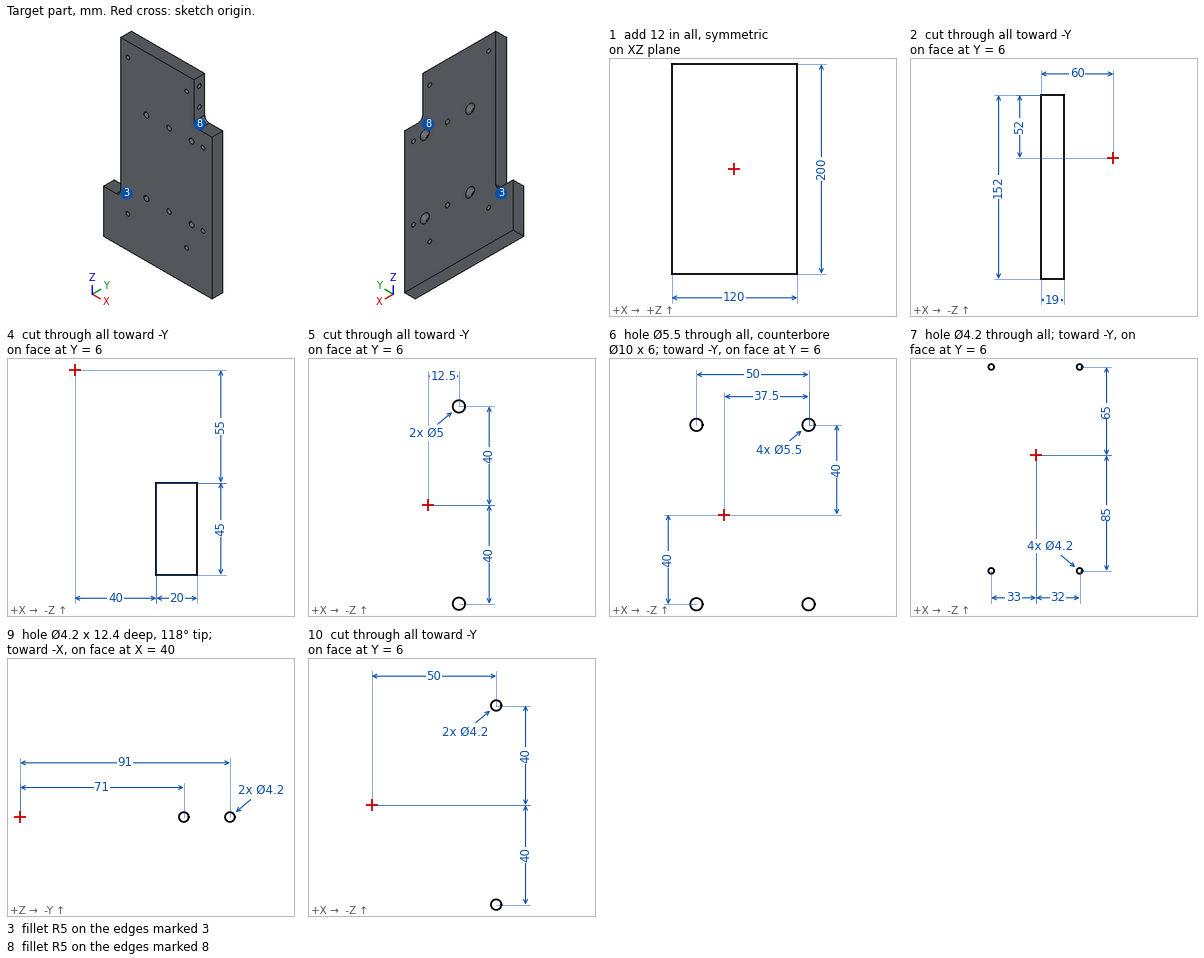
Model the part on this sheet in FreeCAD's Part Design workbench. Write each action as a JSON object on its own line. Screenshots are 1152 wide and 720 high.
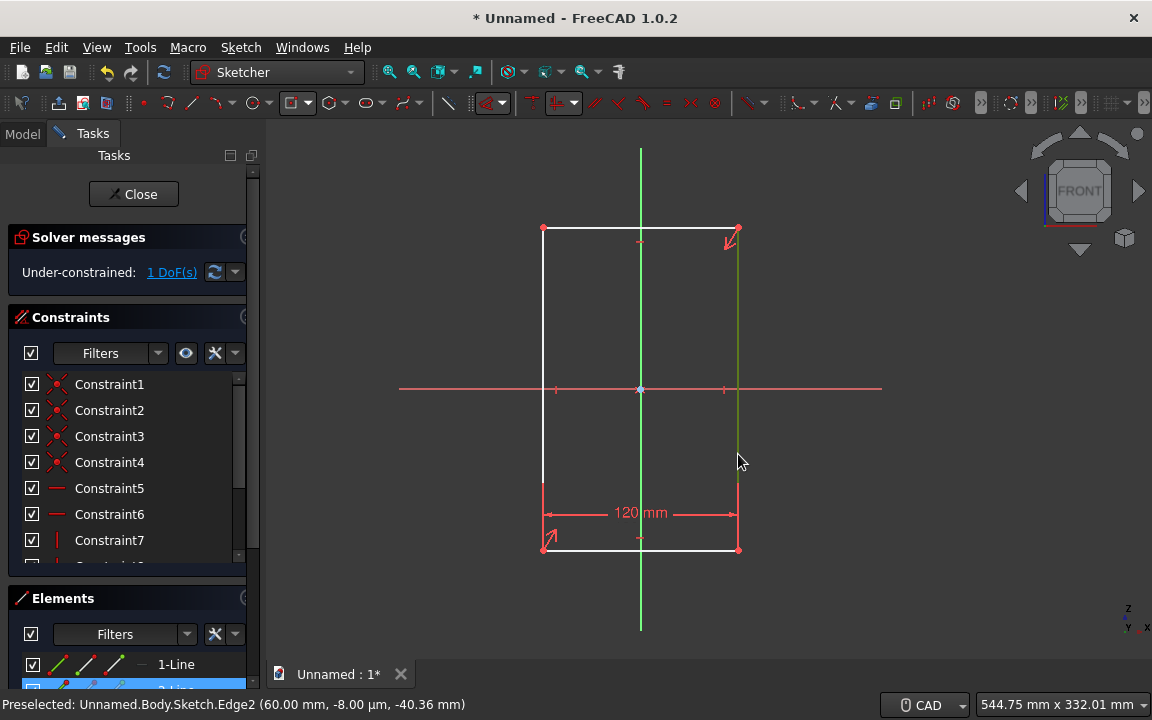
{"action": "key", "text": "i"}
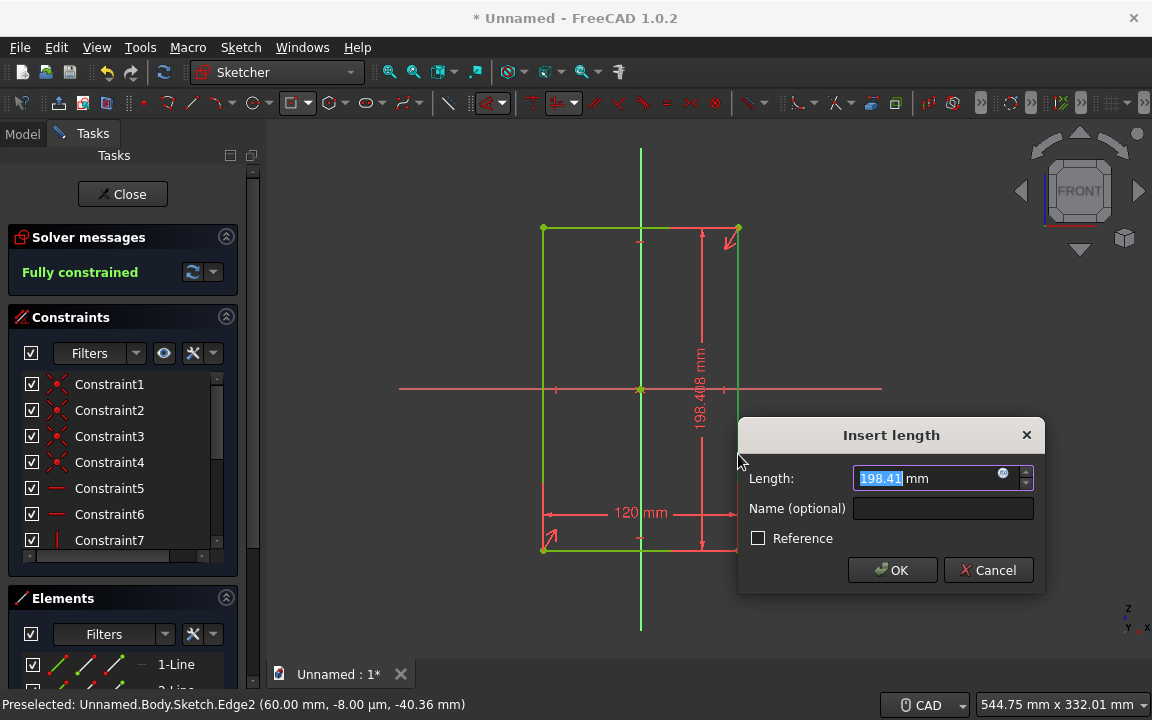
{"action": "type", "text": "200"}
{"action": "key", "text": "Return"}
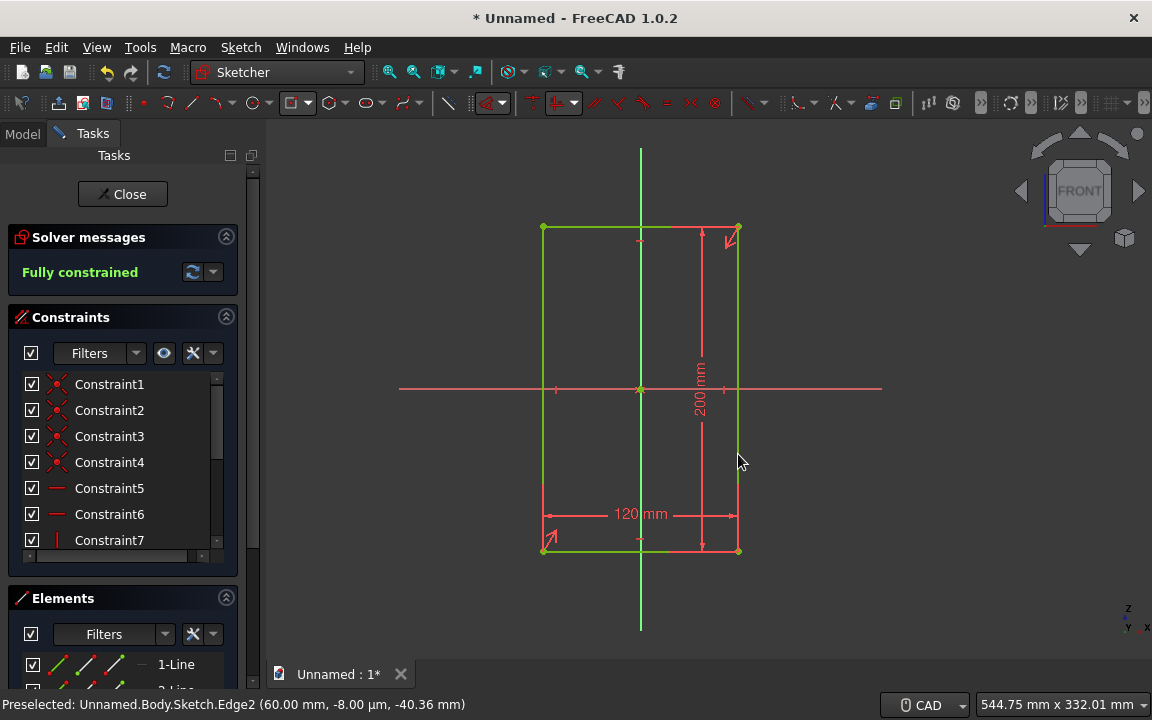
{"action": "left_click", "coordinate": [123, 194]}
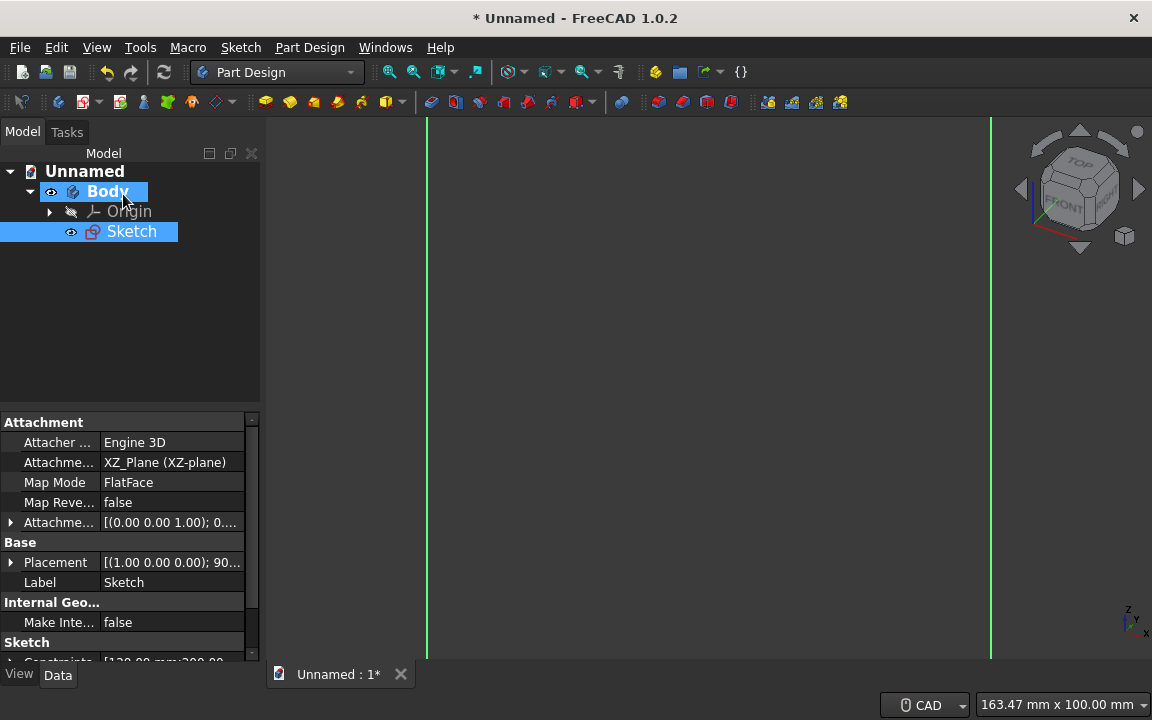
{"action": "left_click", "coordinate": [266, 102]}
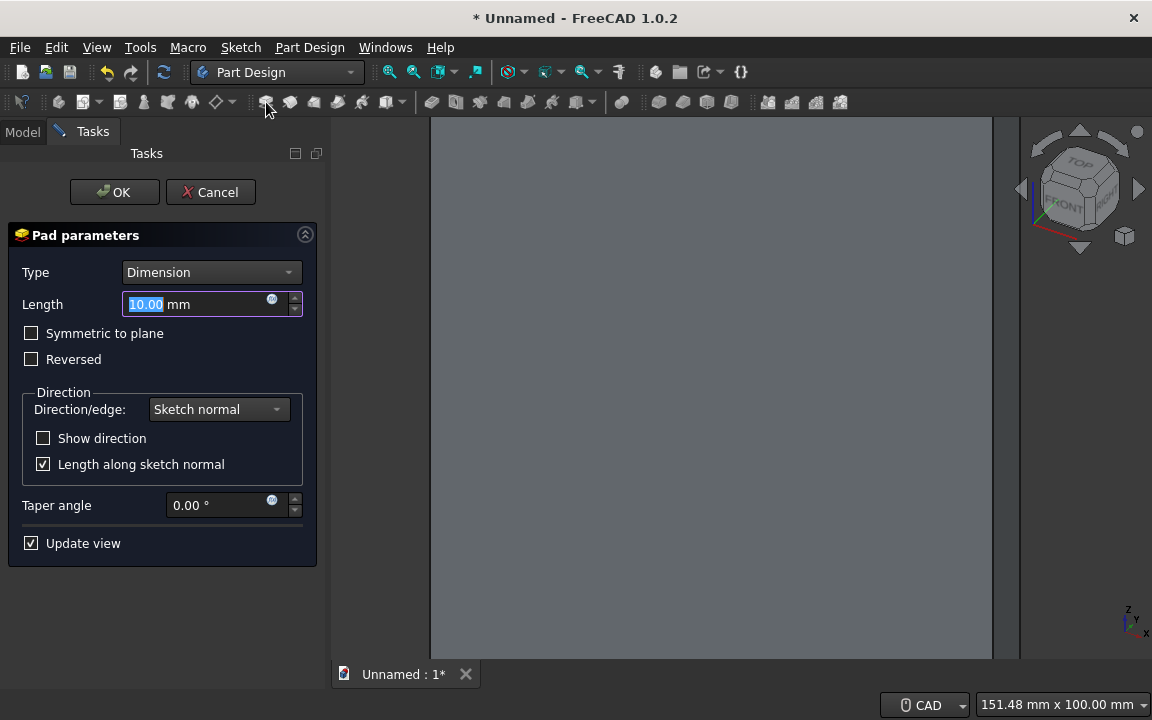
{"action": "type", "text": "12"}
{"action": "key", "text": "Tab"}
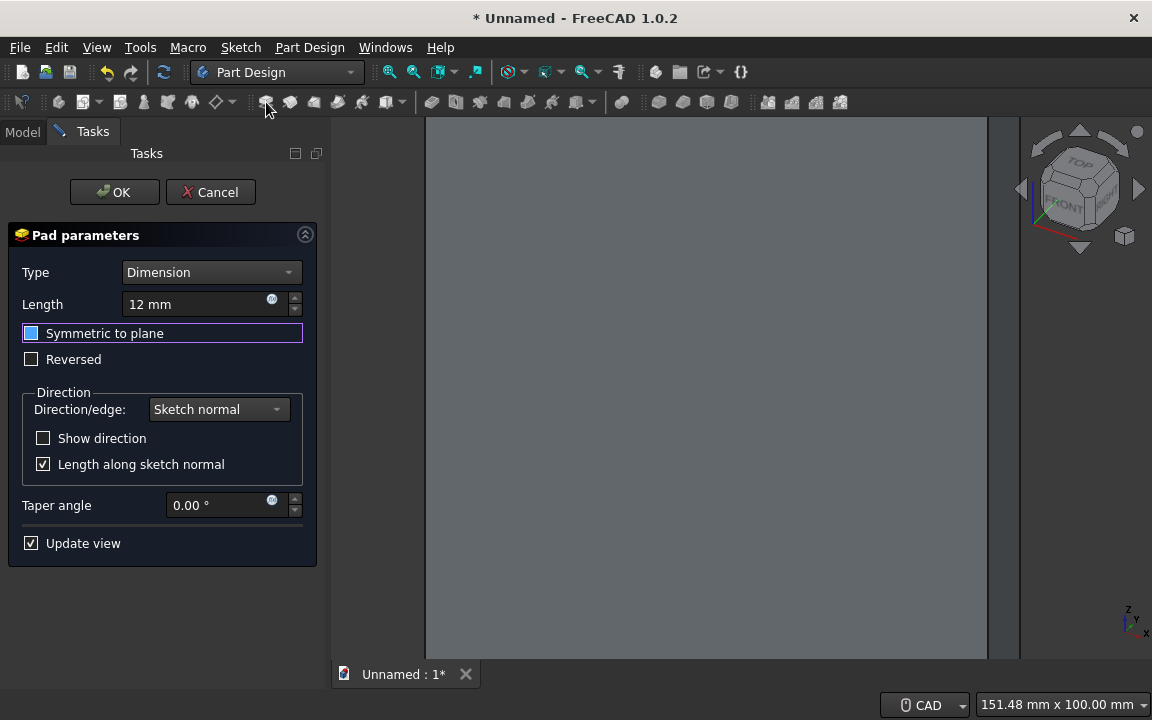
{"action": "left_click", "coordinate": [30, 333]}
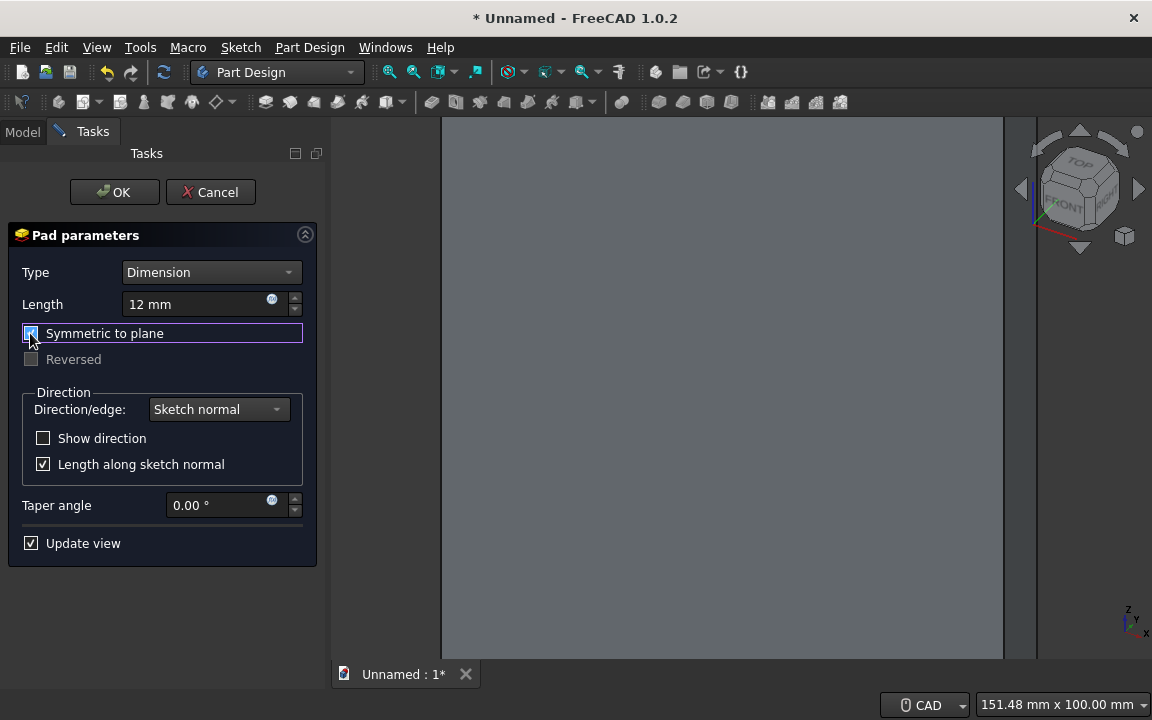
{"action": "left_click", "coordinate": [115, 192]}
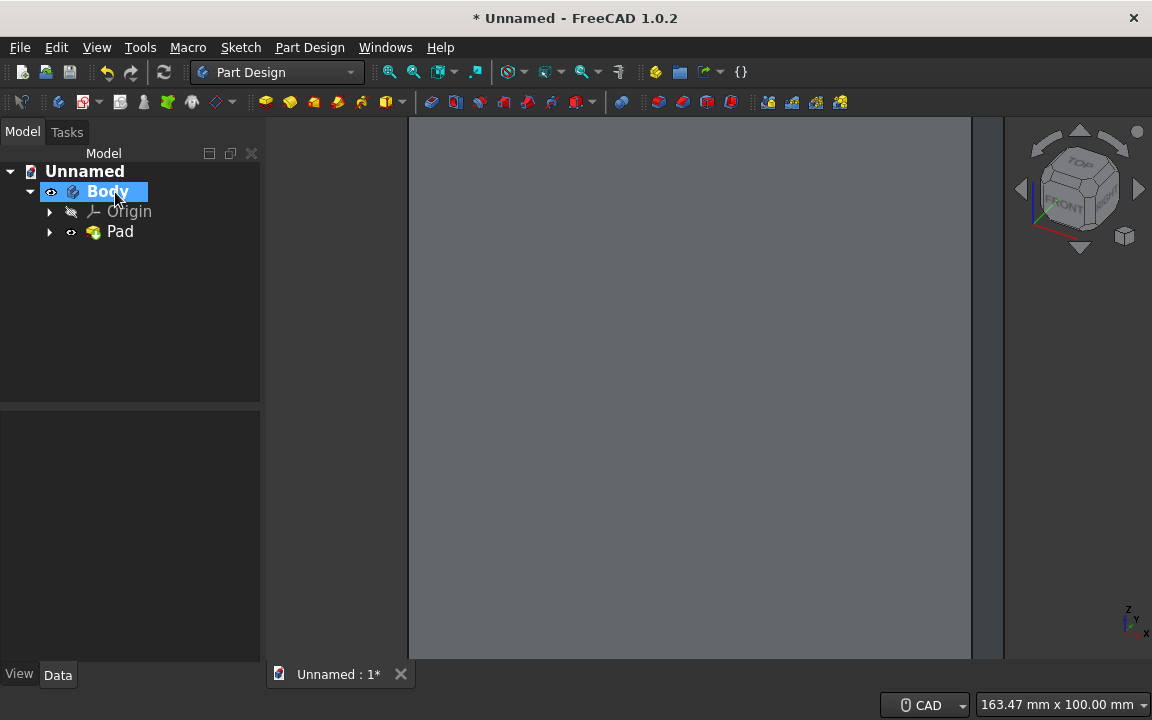
{"action": "left_click", "coordinate": [390, 72]}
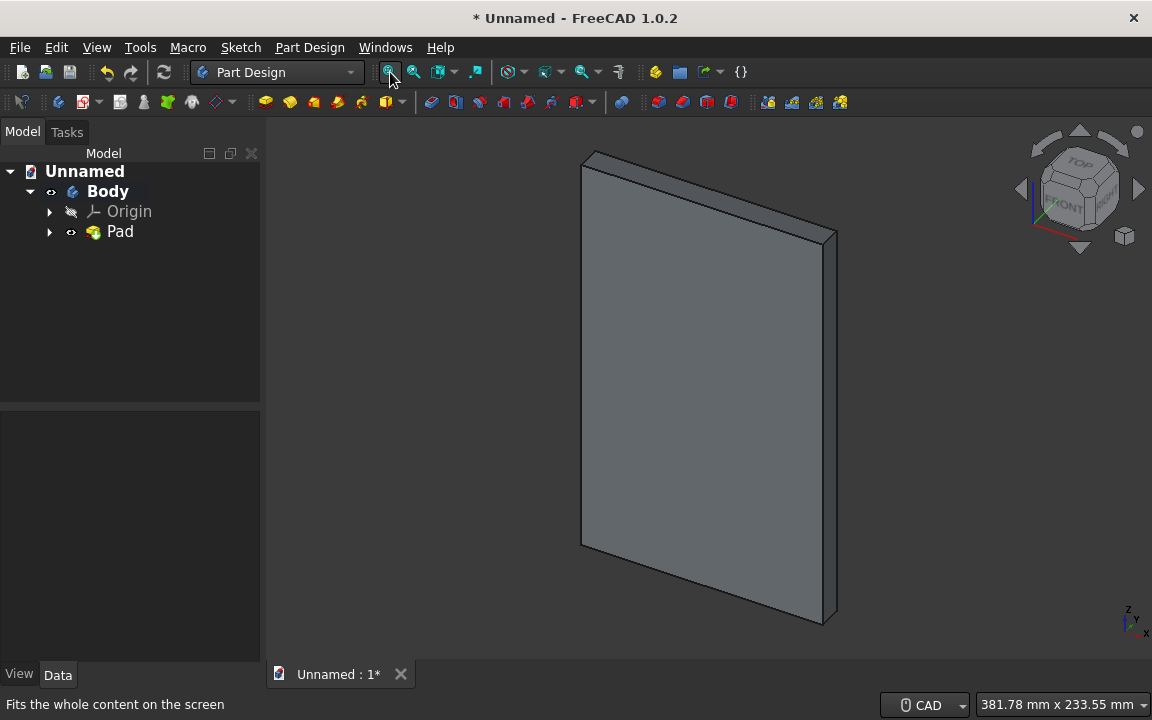
{"action": "key", "text": "4"}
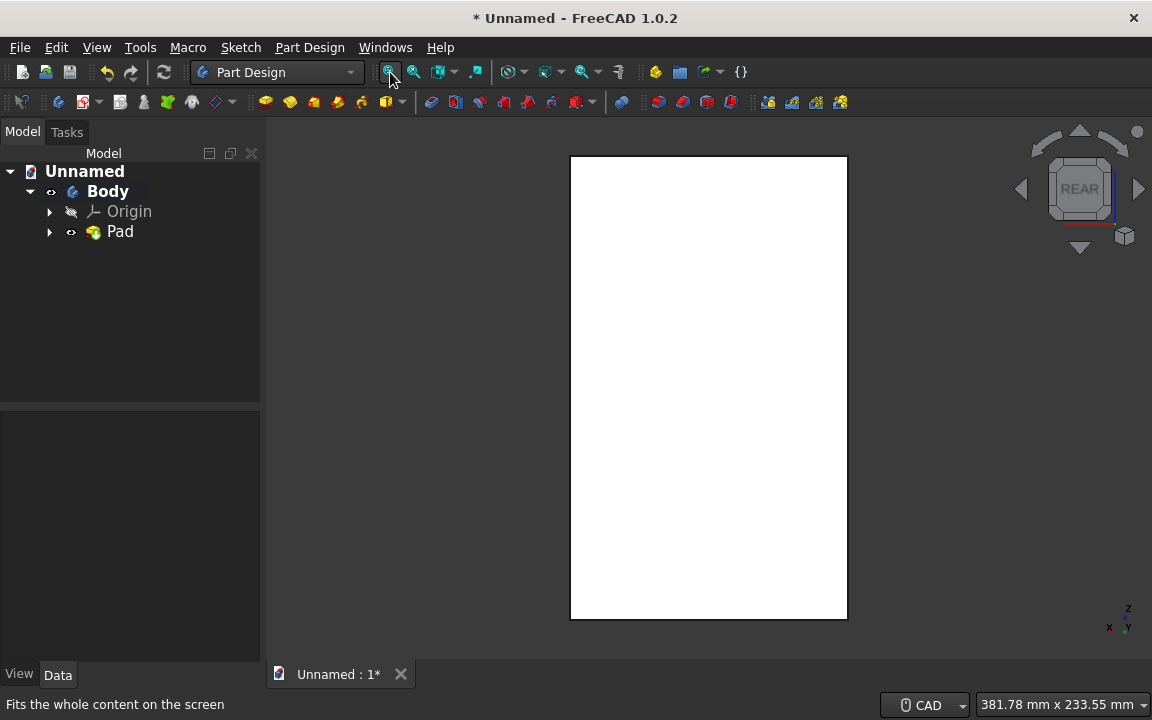
{"action": "left_click", "coordinate": [709, 321]}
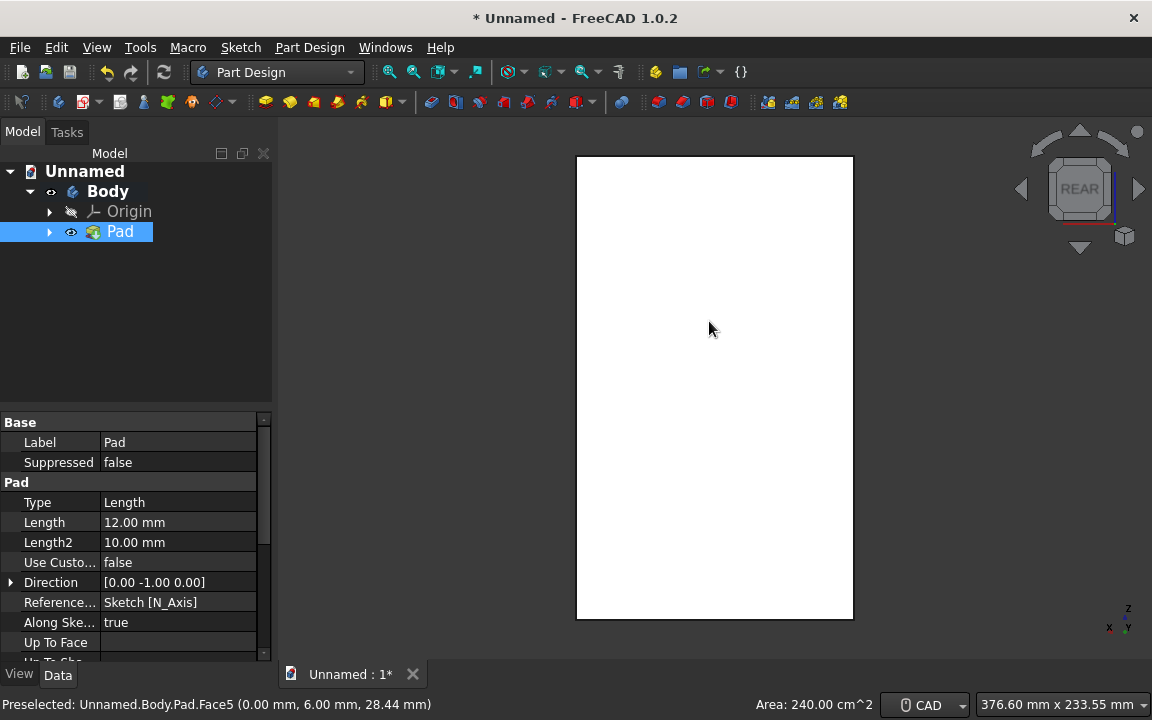
{"action": "left_click", "coordinate": [84, 102]}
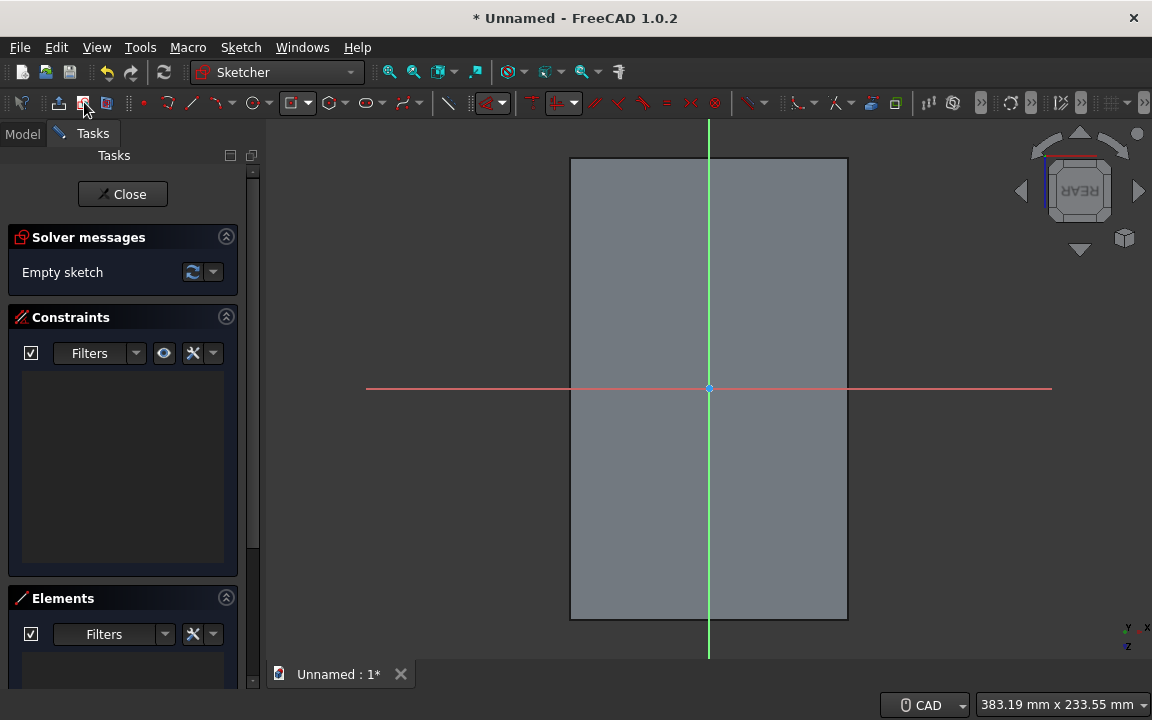
{"action": "scroll", "coordinate": [644, 147], "scroll_direction": "down", "scroll_amount": 1}